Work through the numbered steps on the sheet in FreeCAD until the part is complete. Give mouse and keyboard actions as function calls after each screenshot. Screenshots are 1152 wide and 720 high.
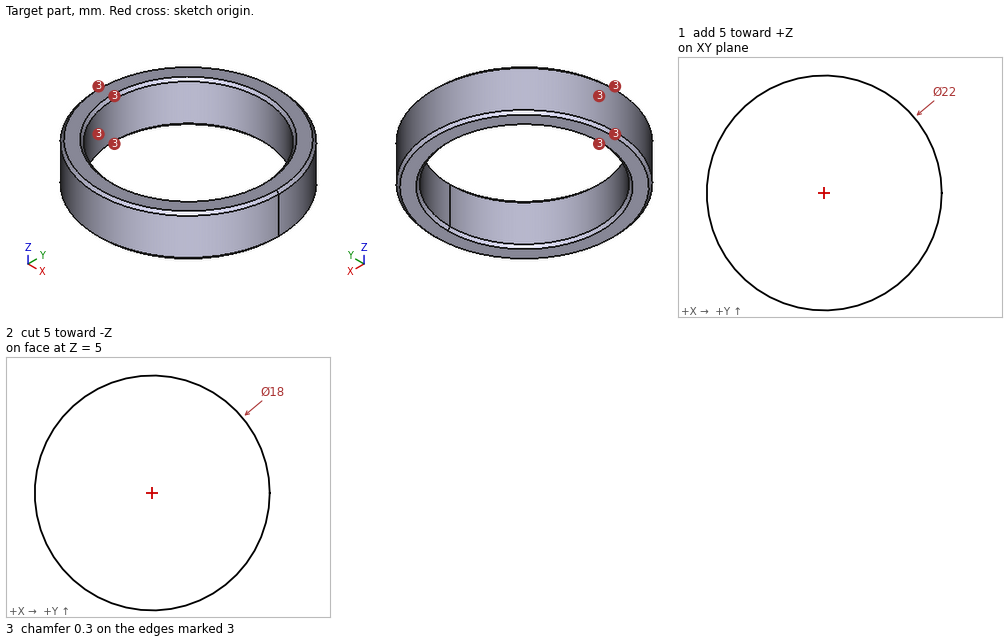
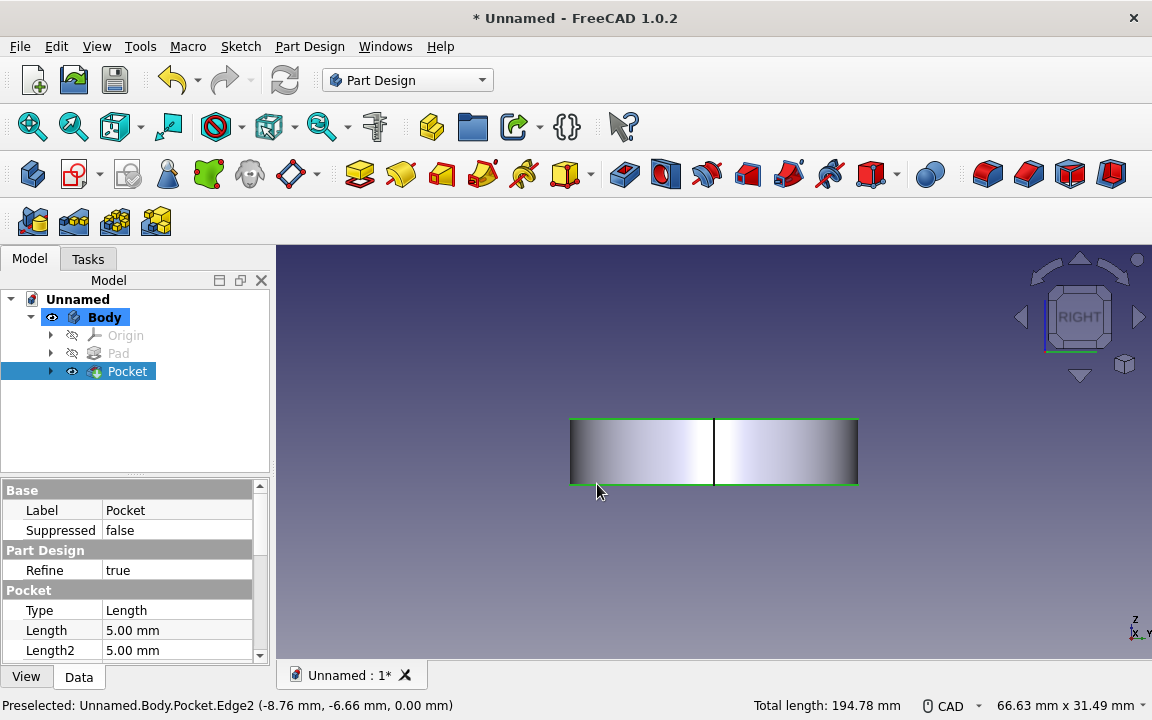
click(33, 128)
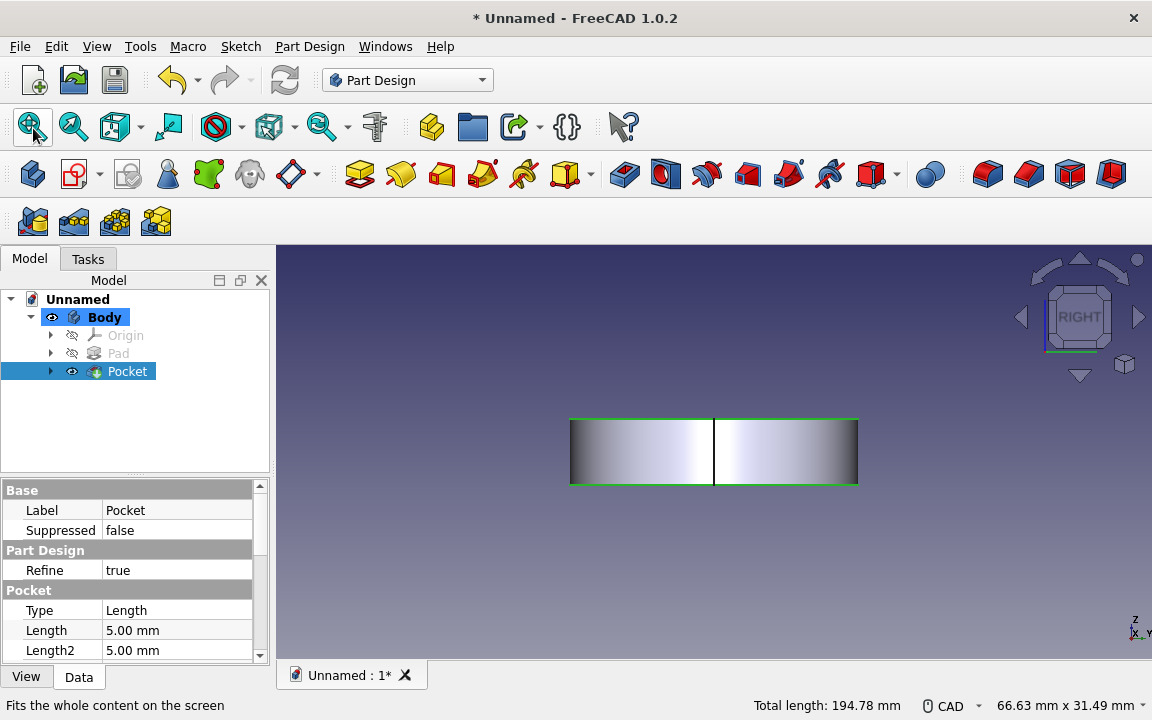
key(5)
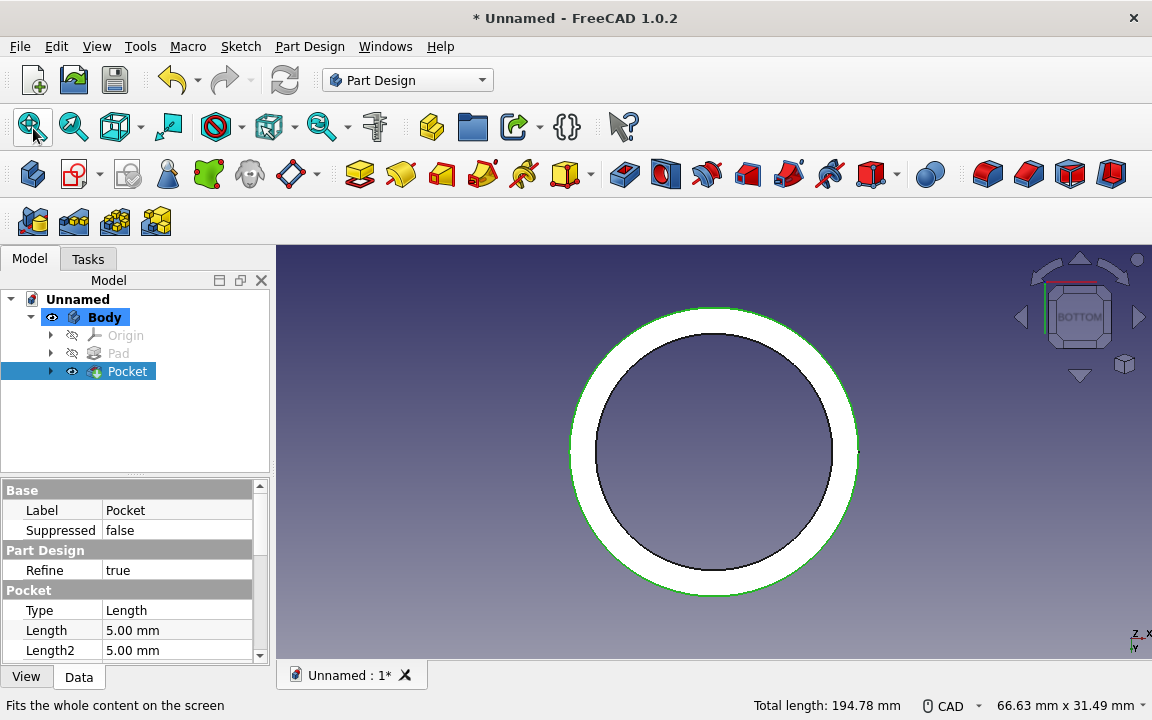
click(596, 451, ctrl)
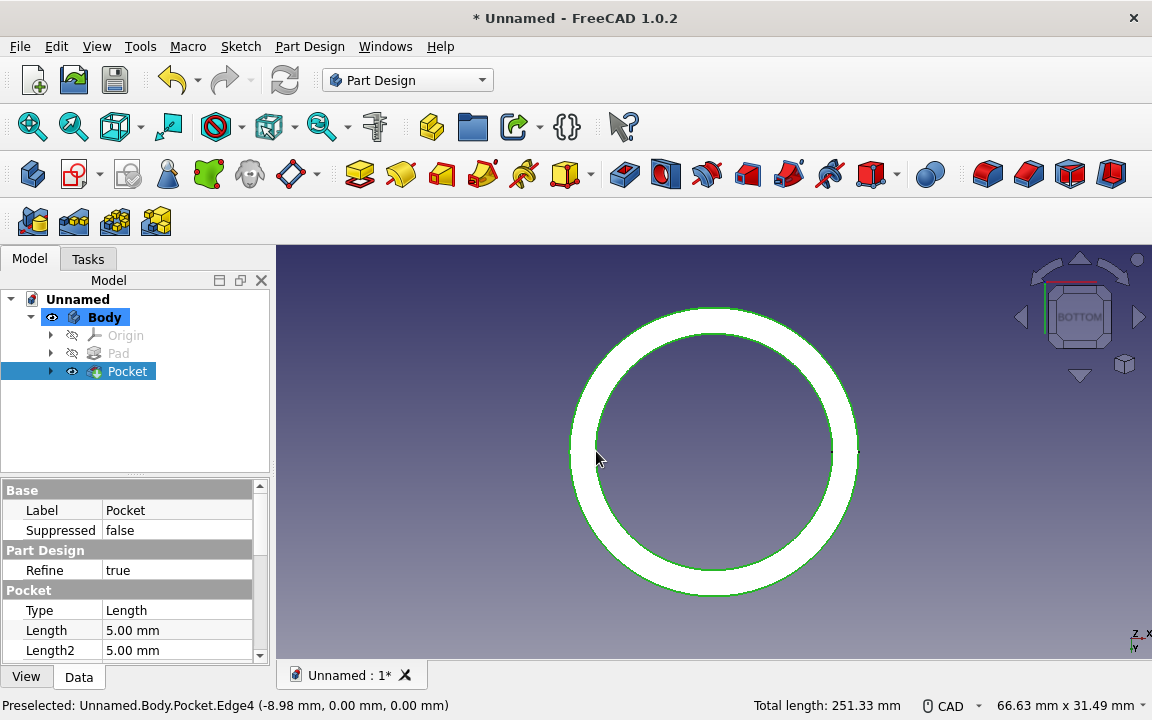
click(1029, 174)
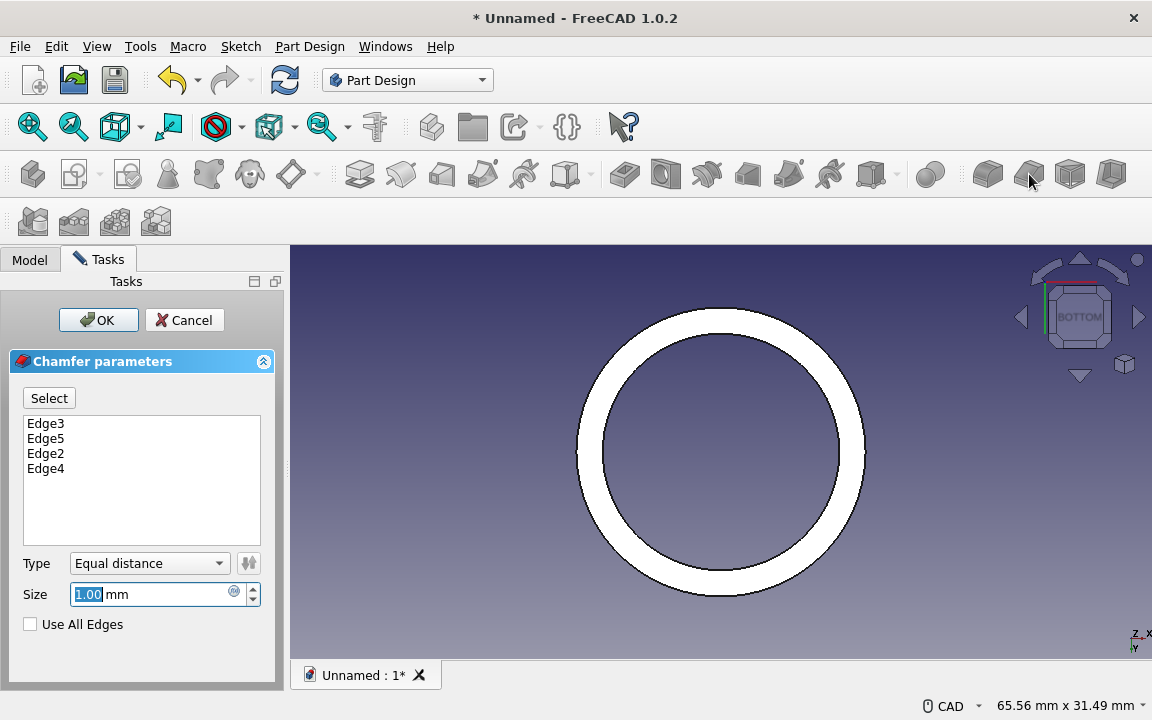
text(0.3)
key(Tab)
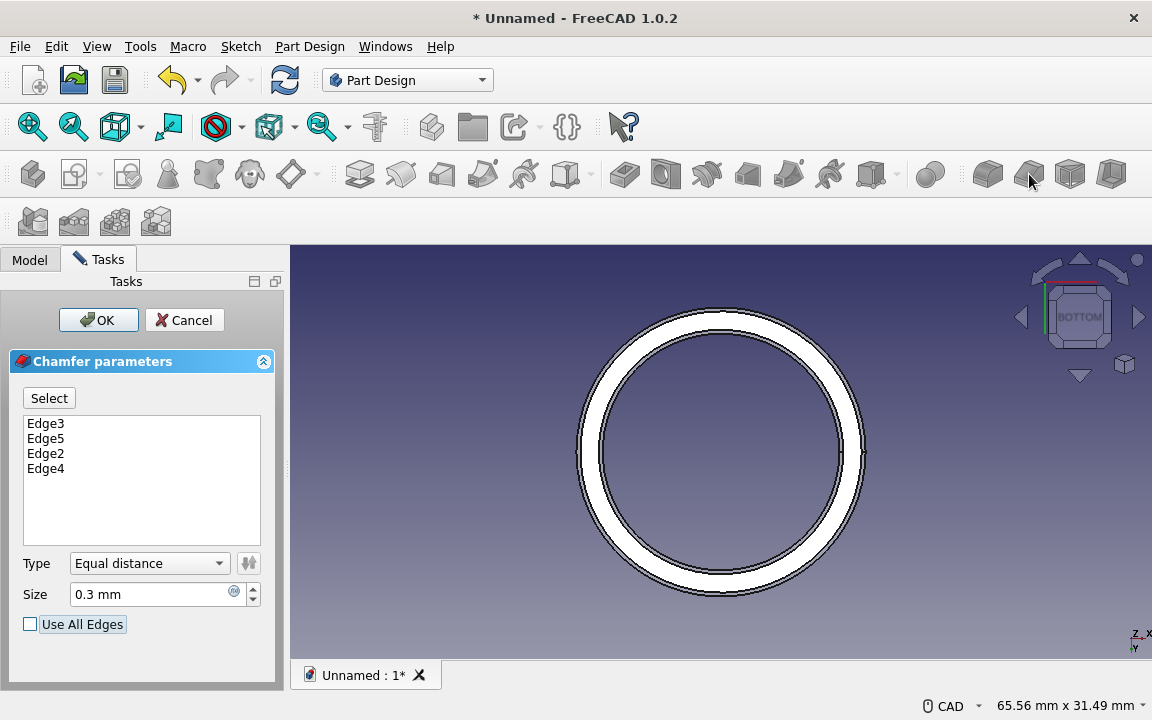
click(99, 320)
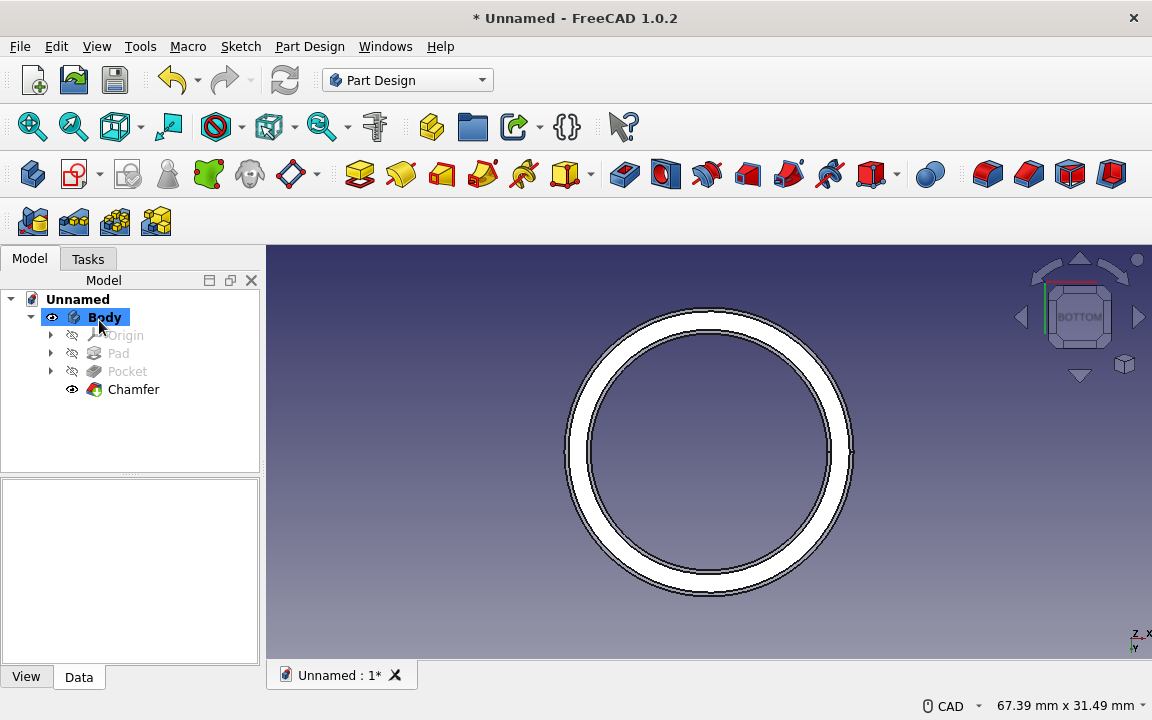
key(0)